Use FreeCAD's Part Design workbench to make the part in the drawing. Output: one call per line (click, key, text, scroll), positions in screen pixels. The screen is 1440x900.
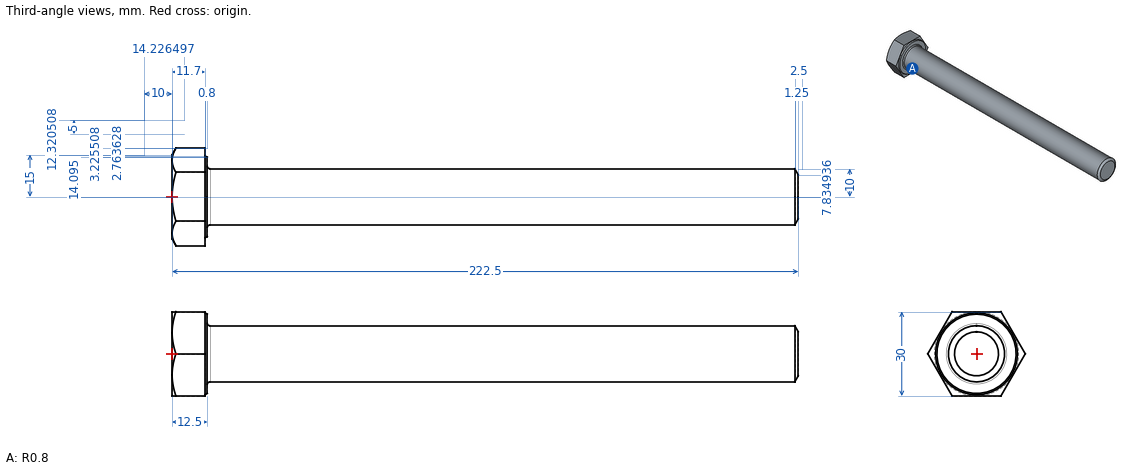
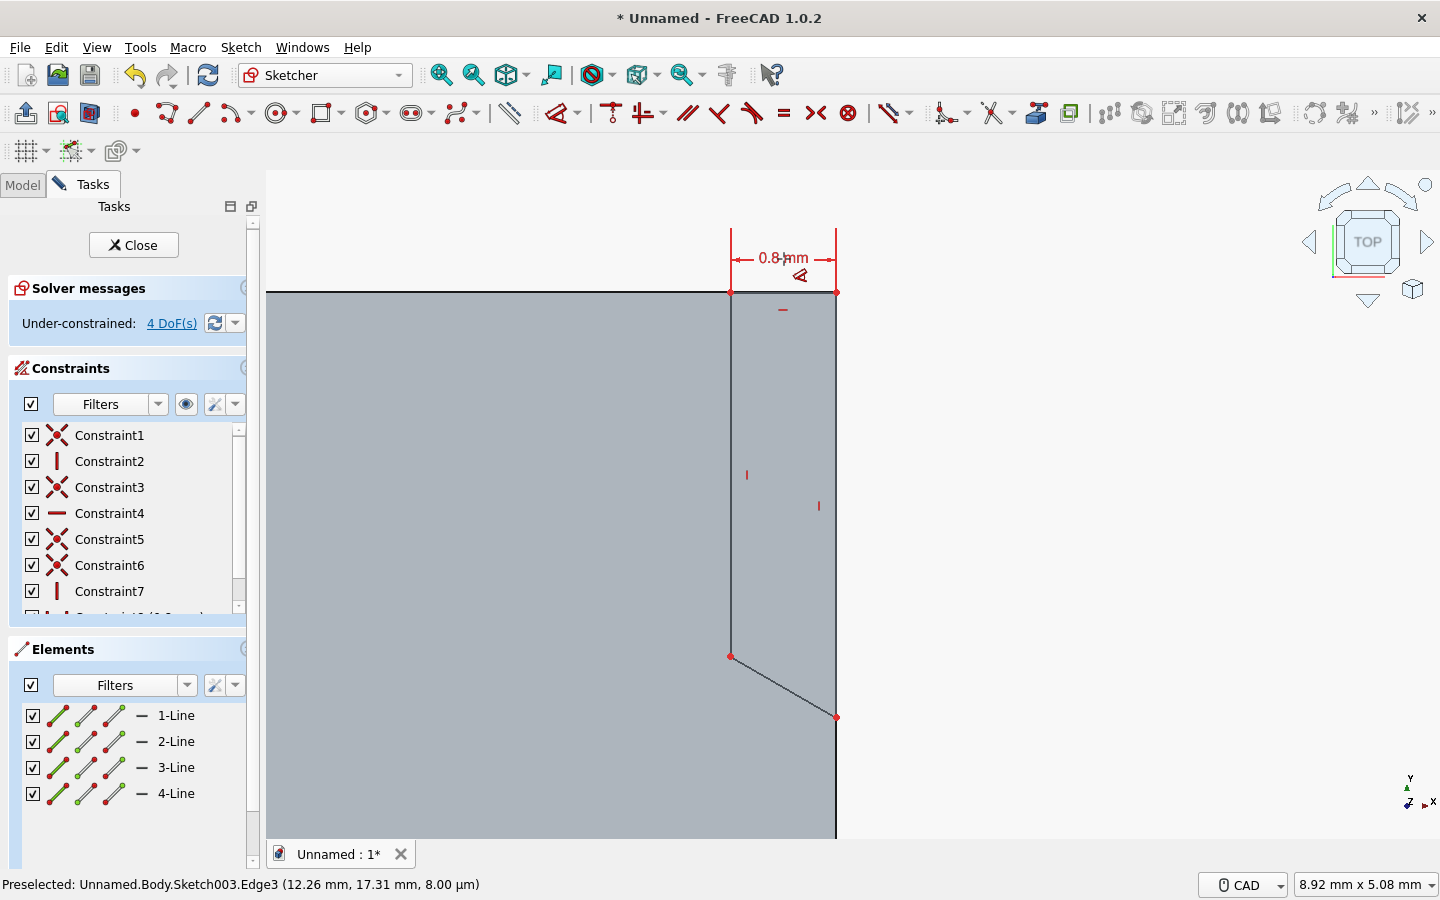
click(731, 657)
click(512, 623)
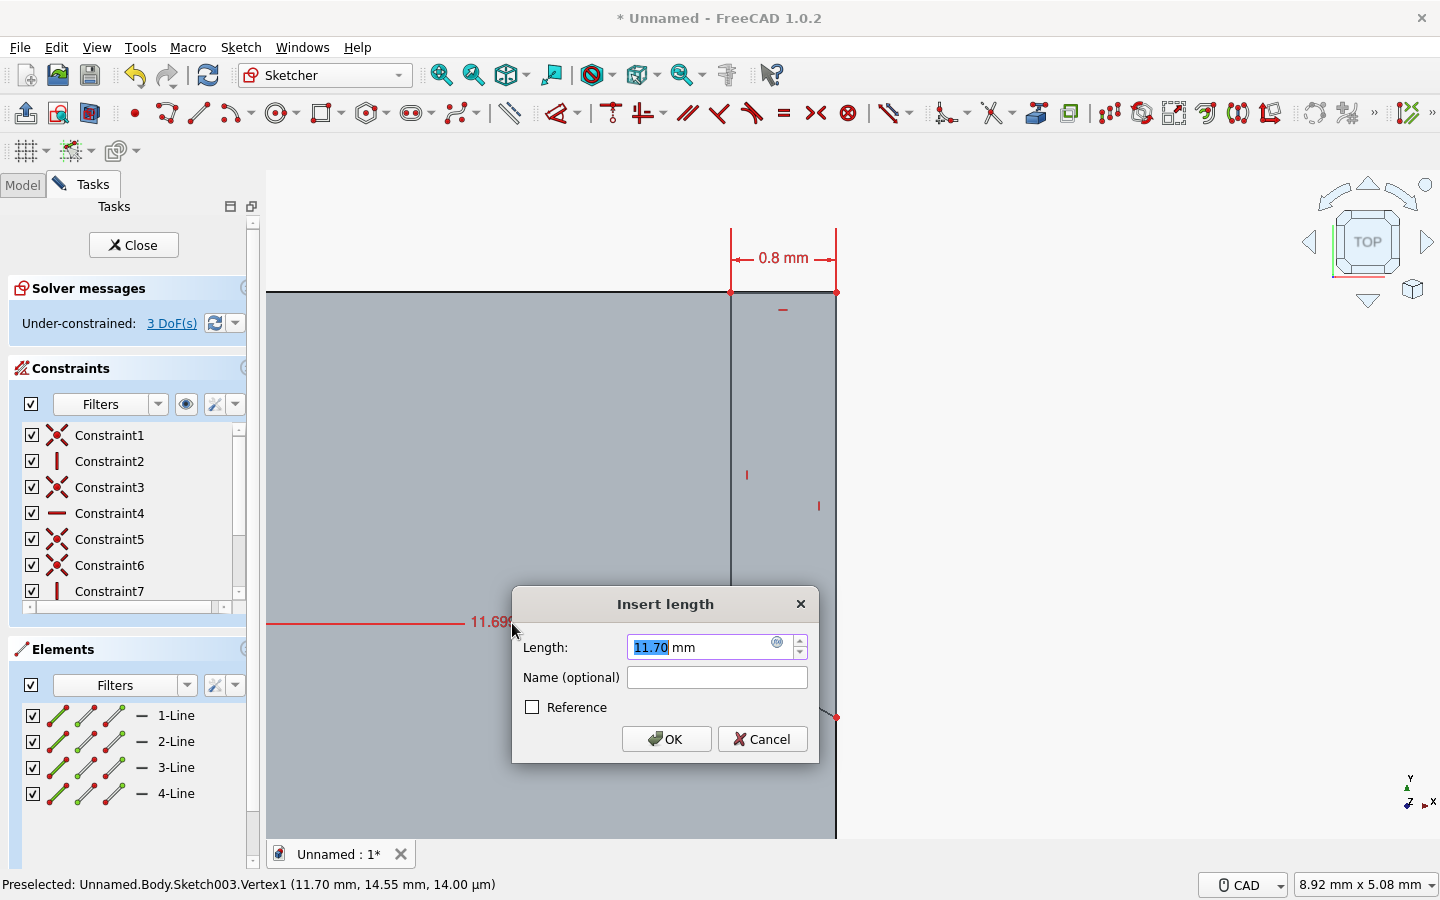
text(11.7)
key(Return)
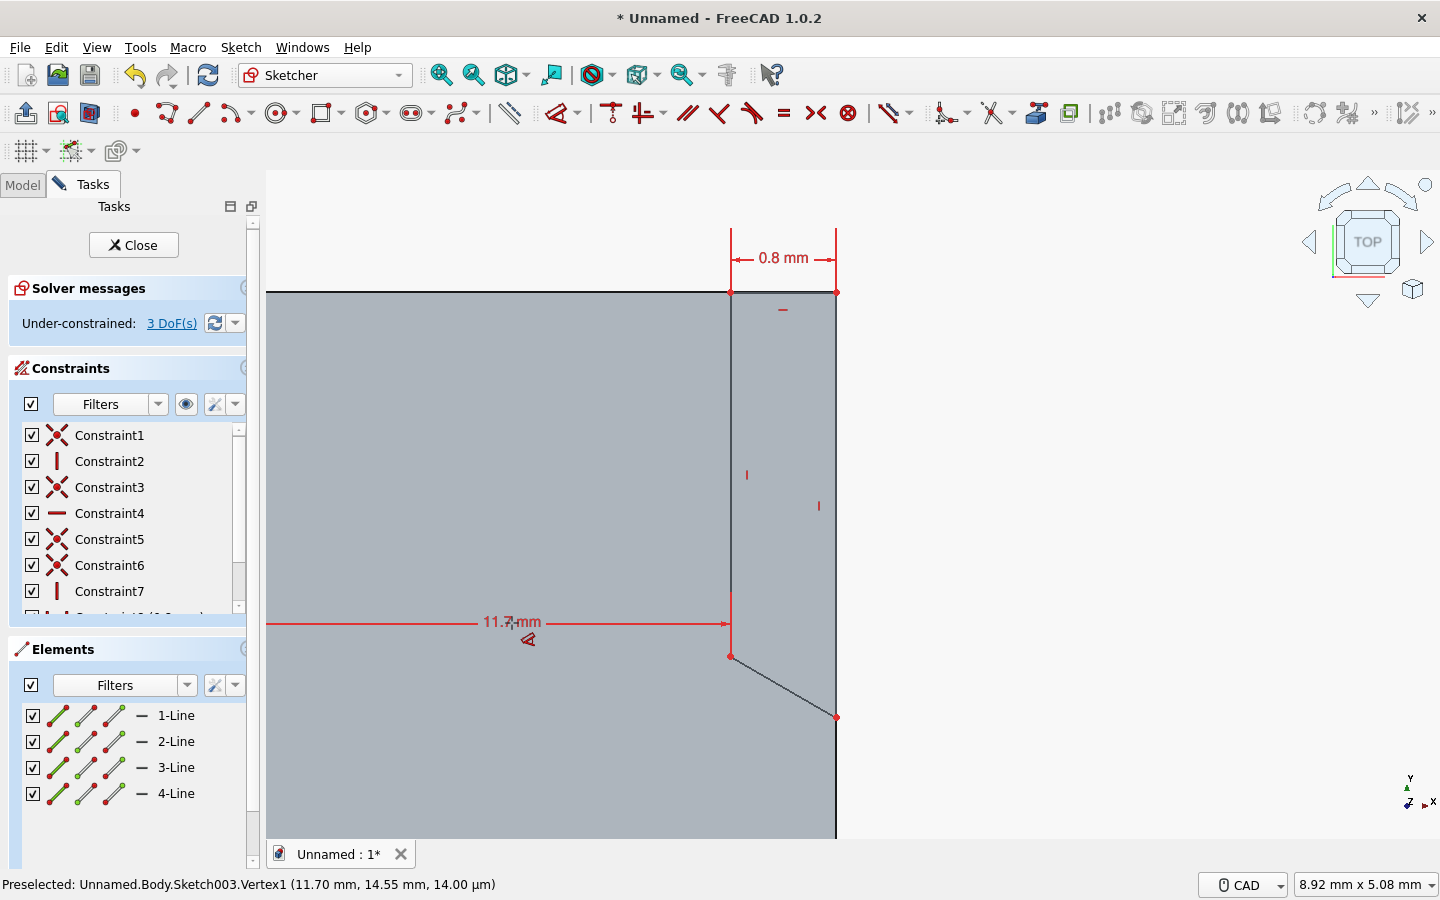
click(836, 718)
click(870, 765)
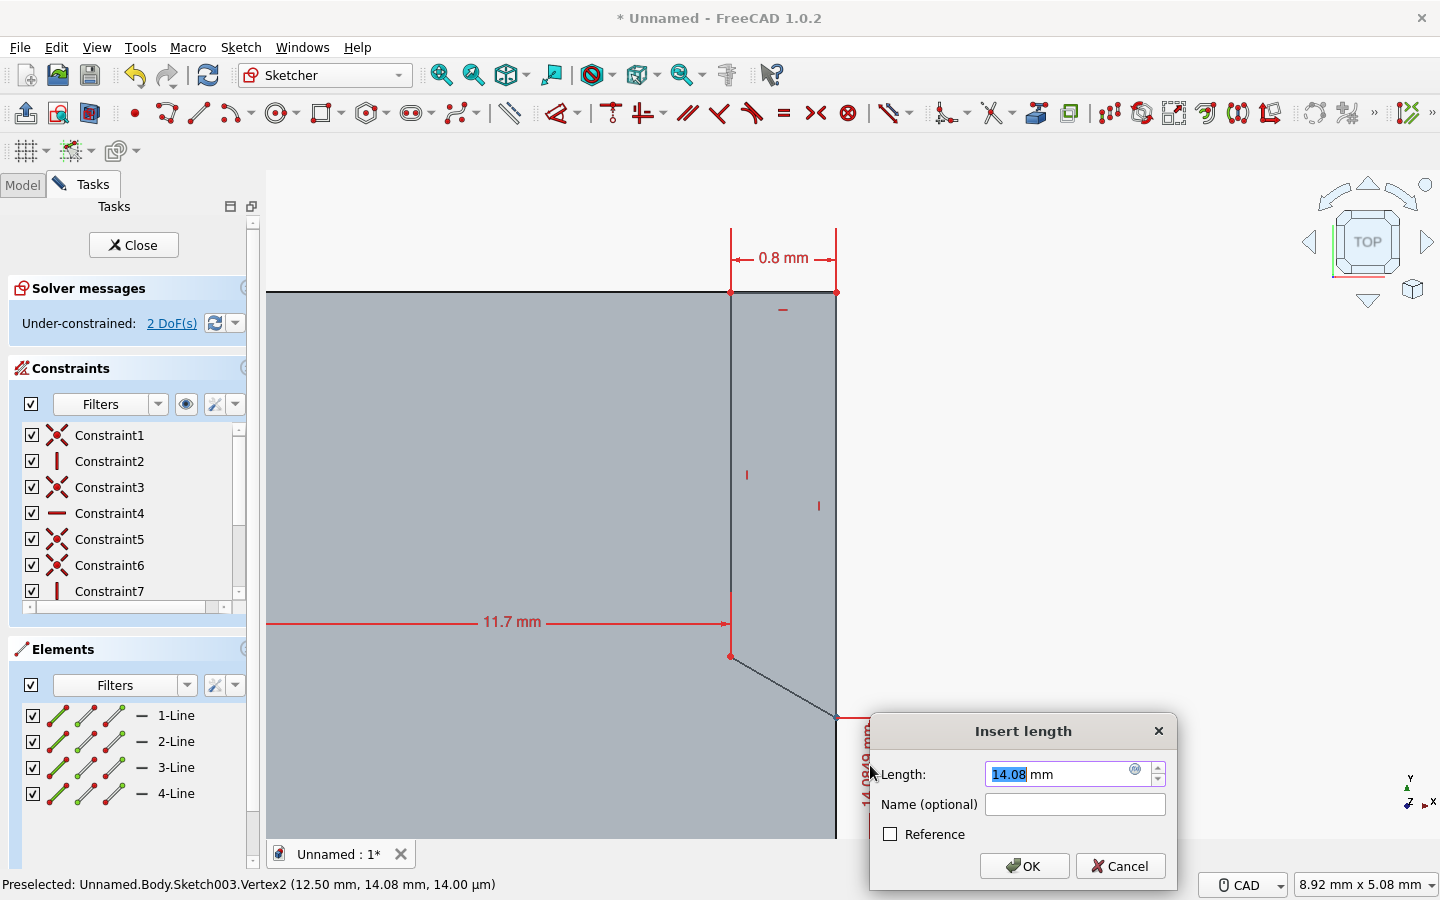
text(14.095)
key(Return)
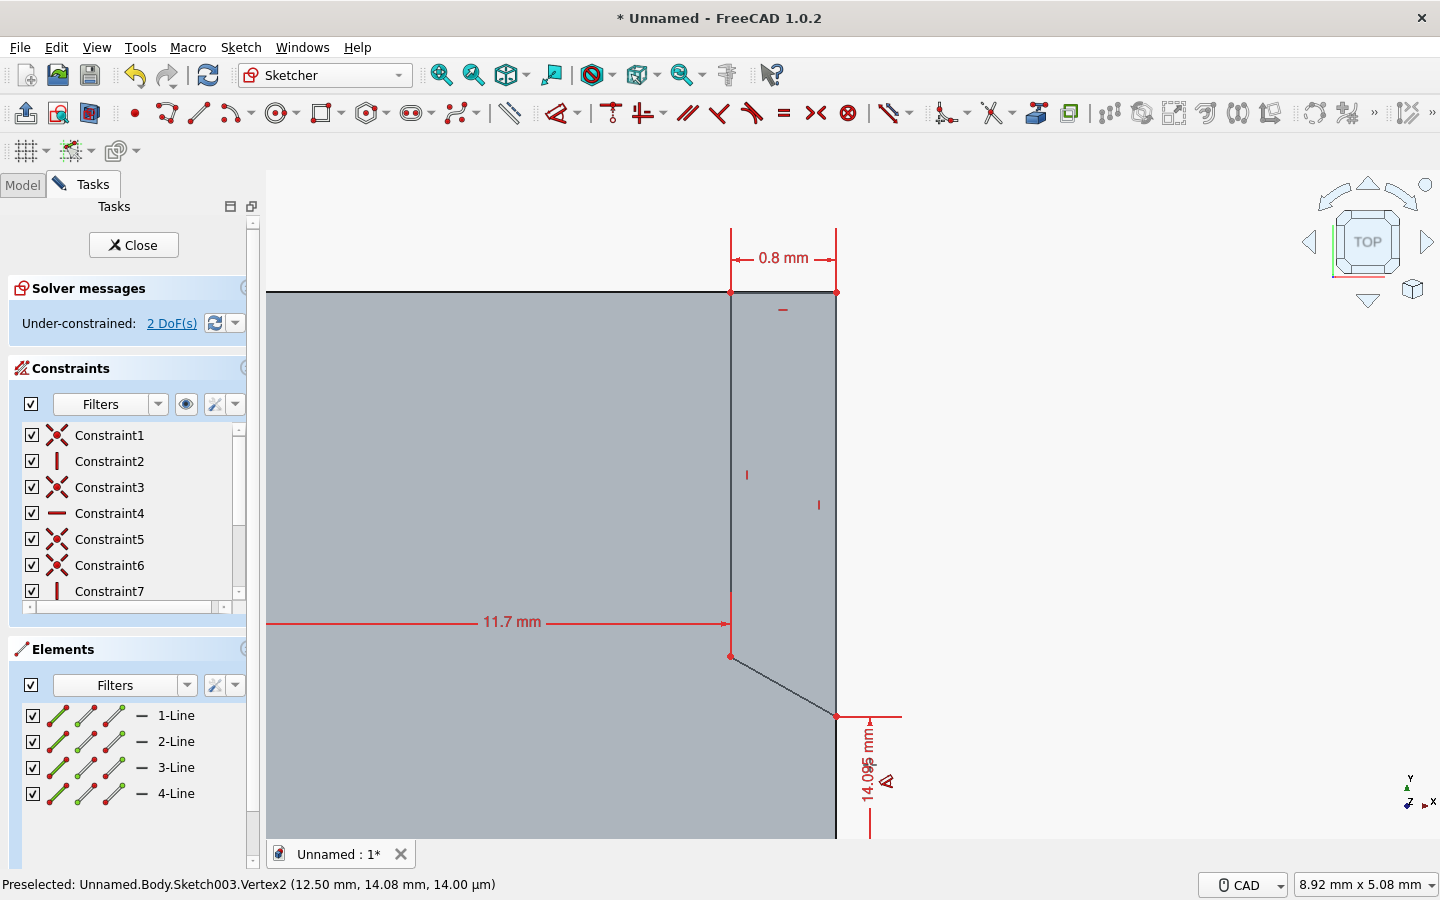
click(836, 590)
click(870, 505)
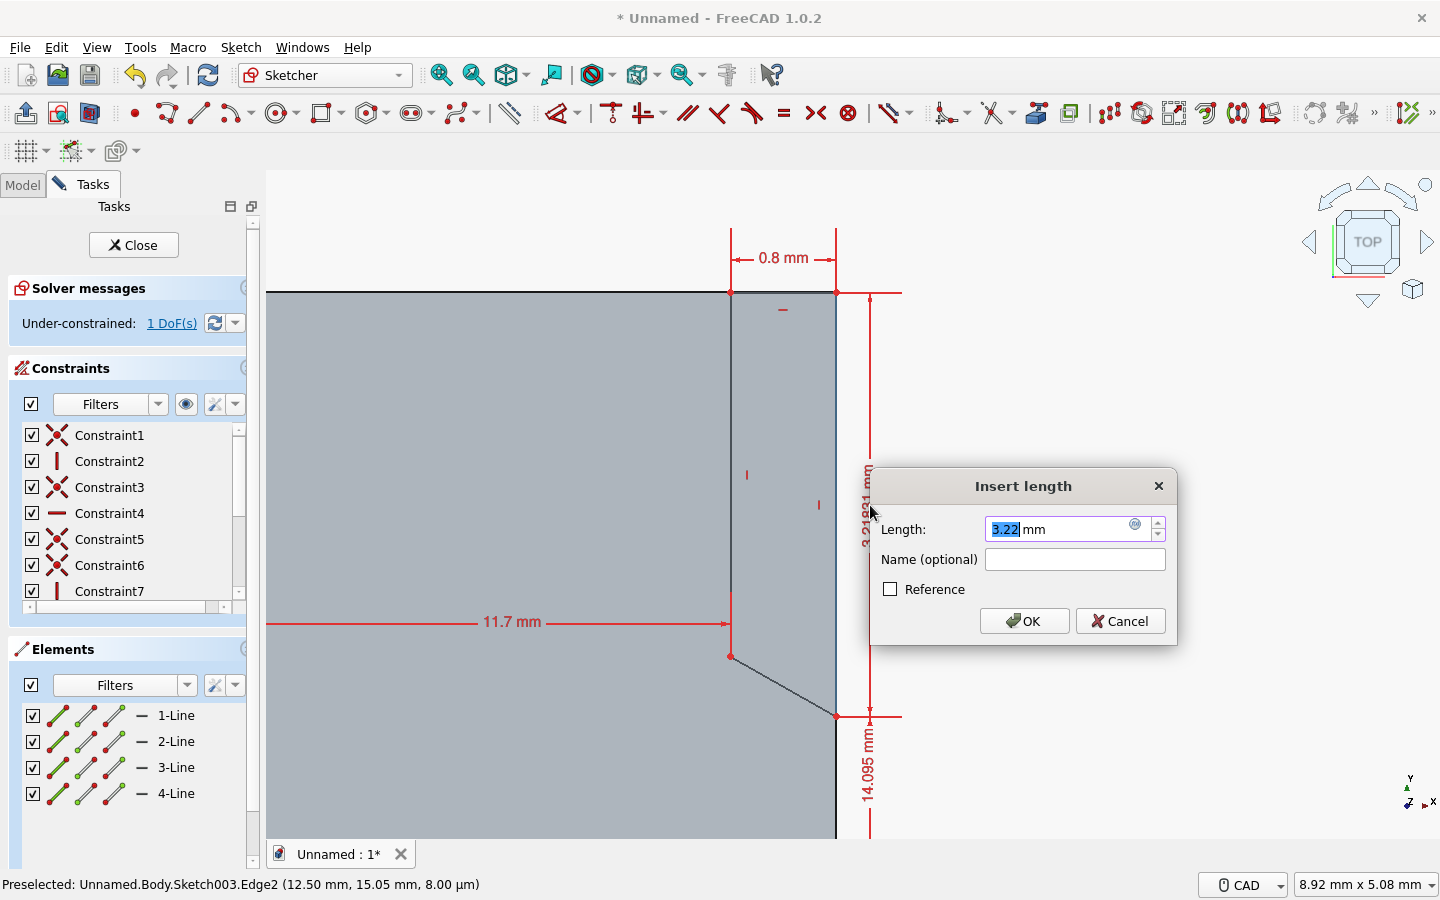
text(3.225508)
key(Return)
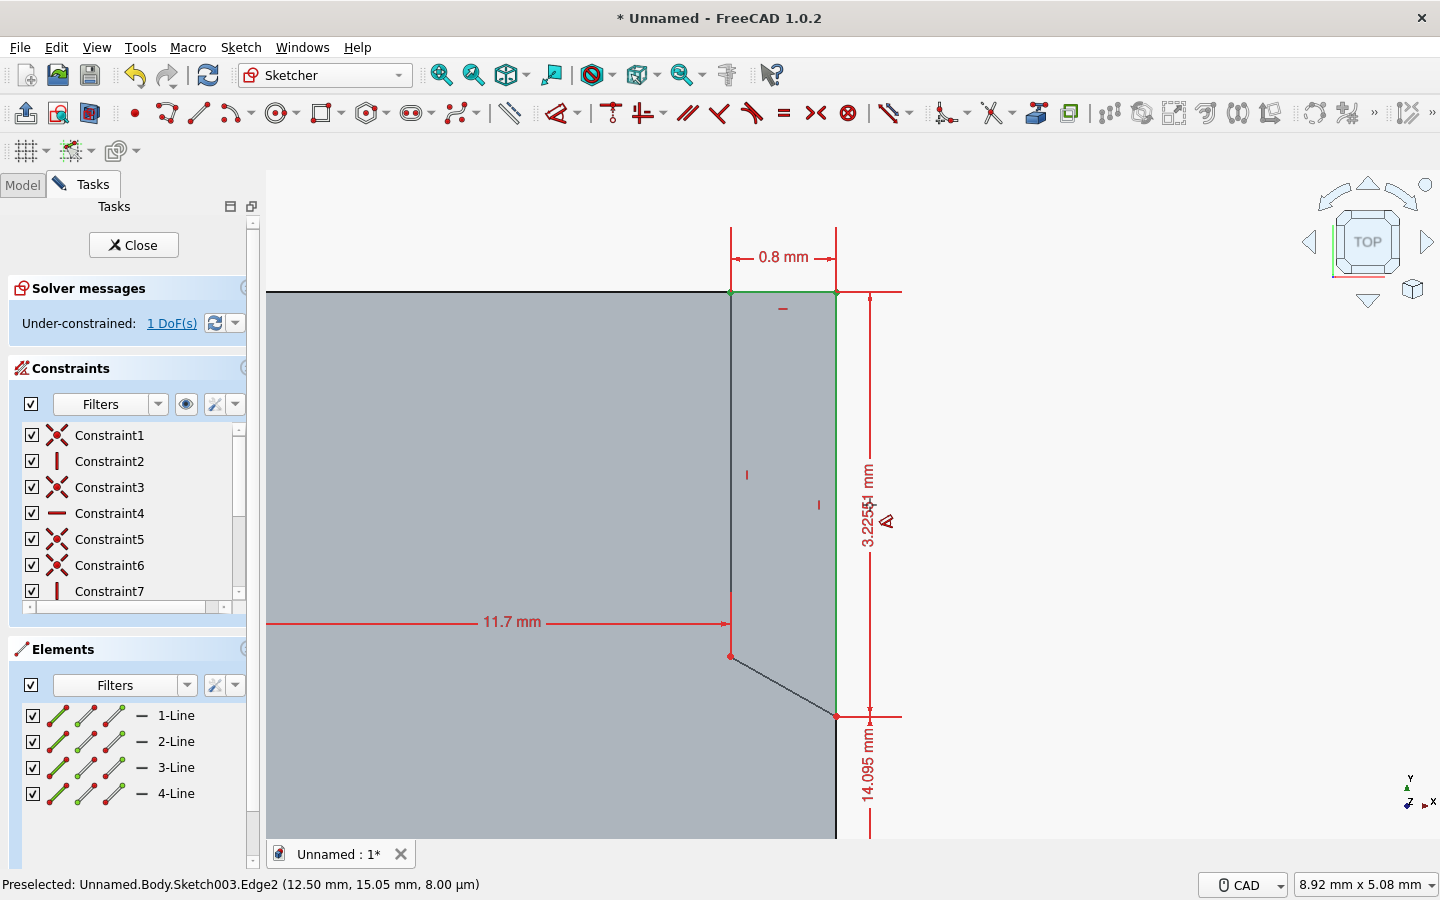
click(731, 402)
click(697, 475)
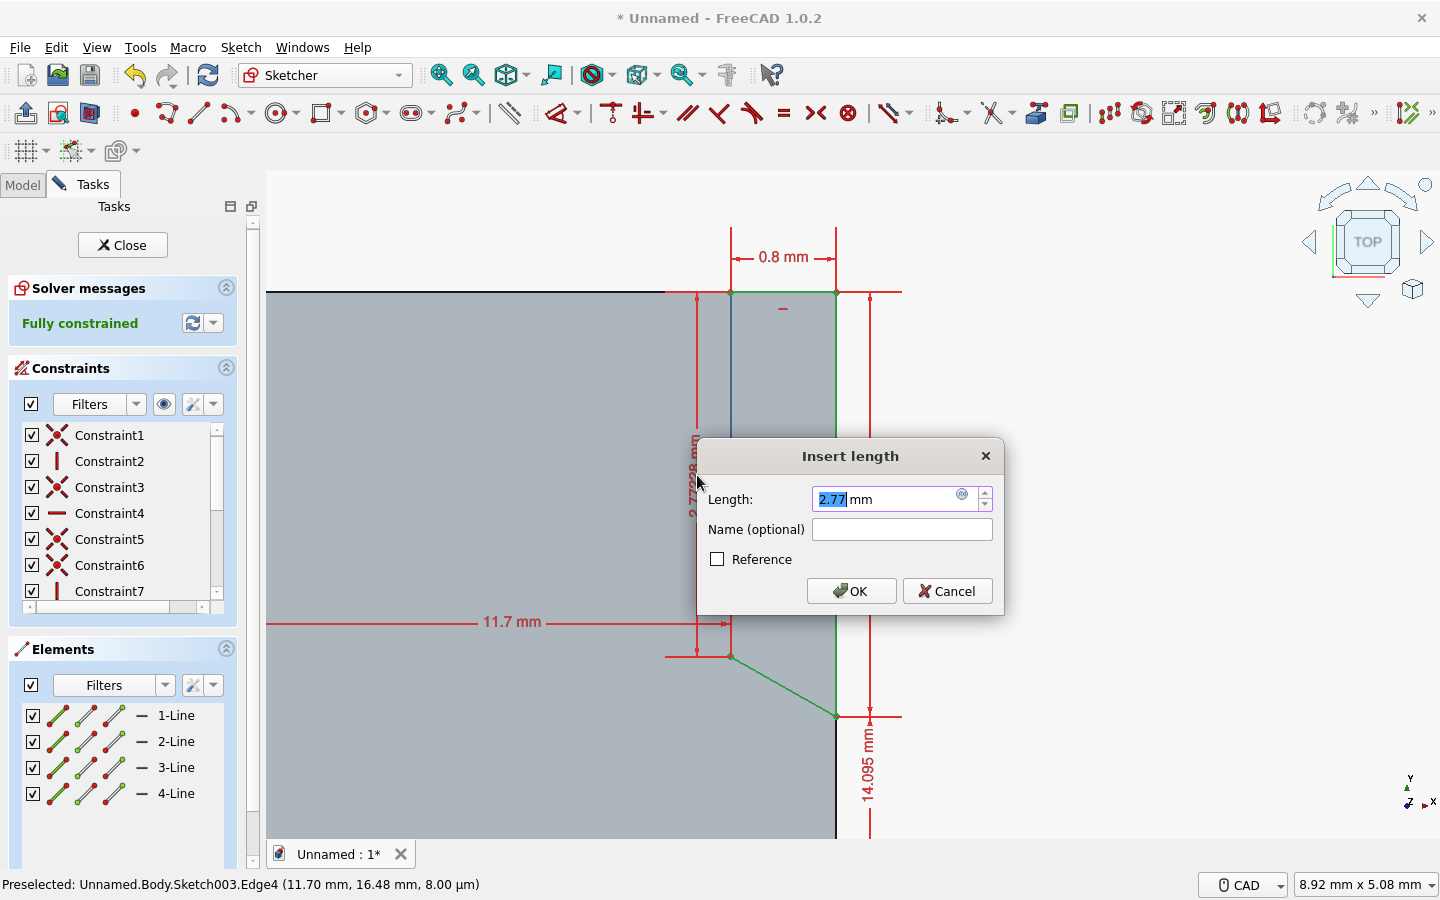
text(2.763628)
key(Return)
key(Escape)